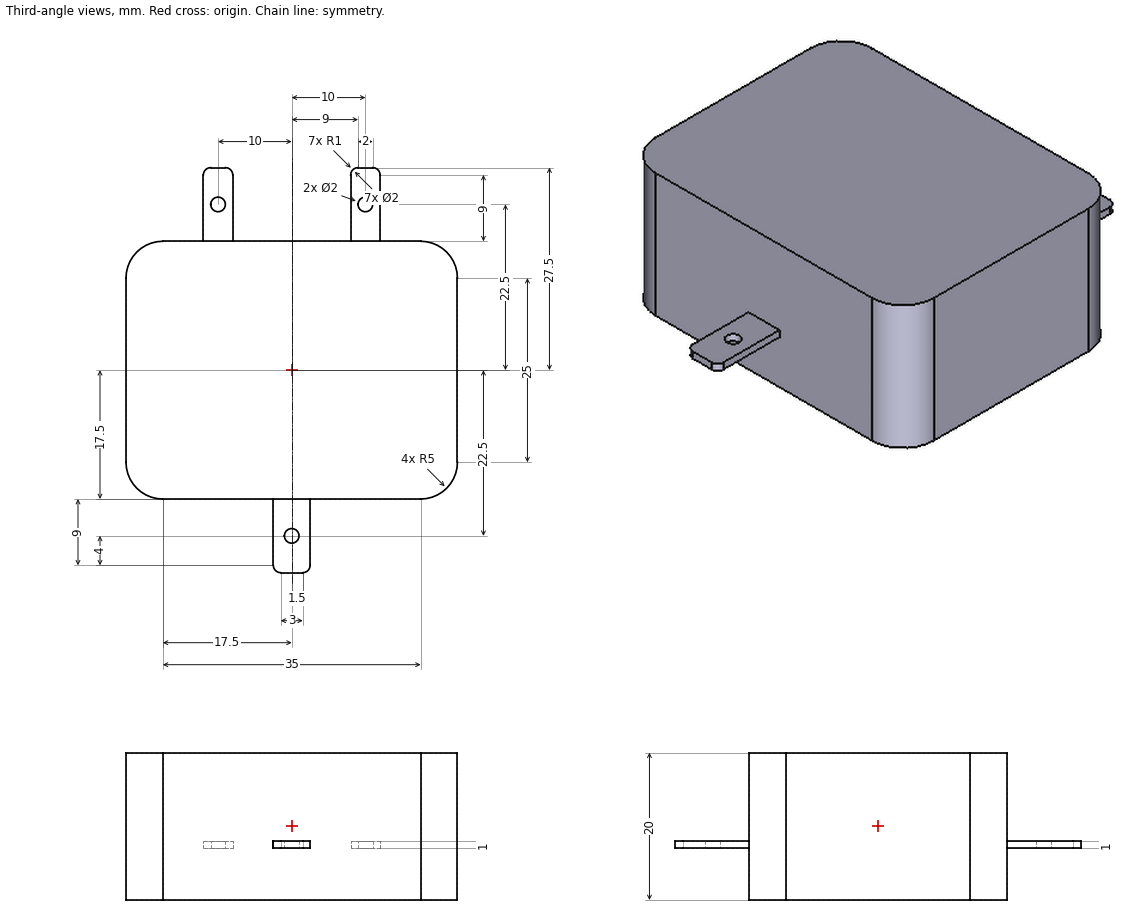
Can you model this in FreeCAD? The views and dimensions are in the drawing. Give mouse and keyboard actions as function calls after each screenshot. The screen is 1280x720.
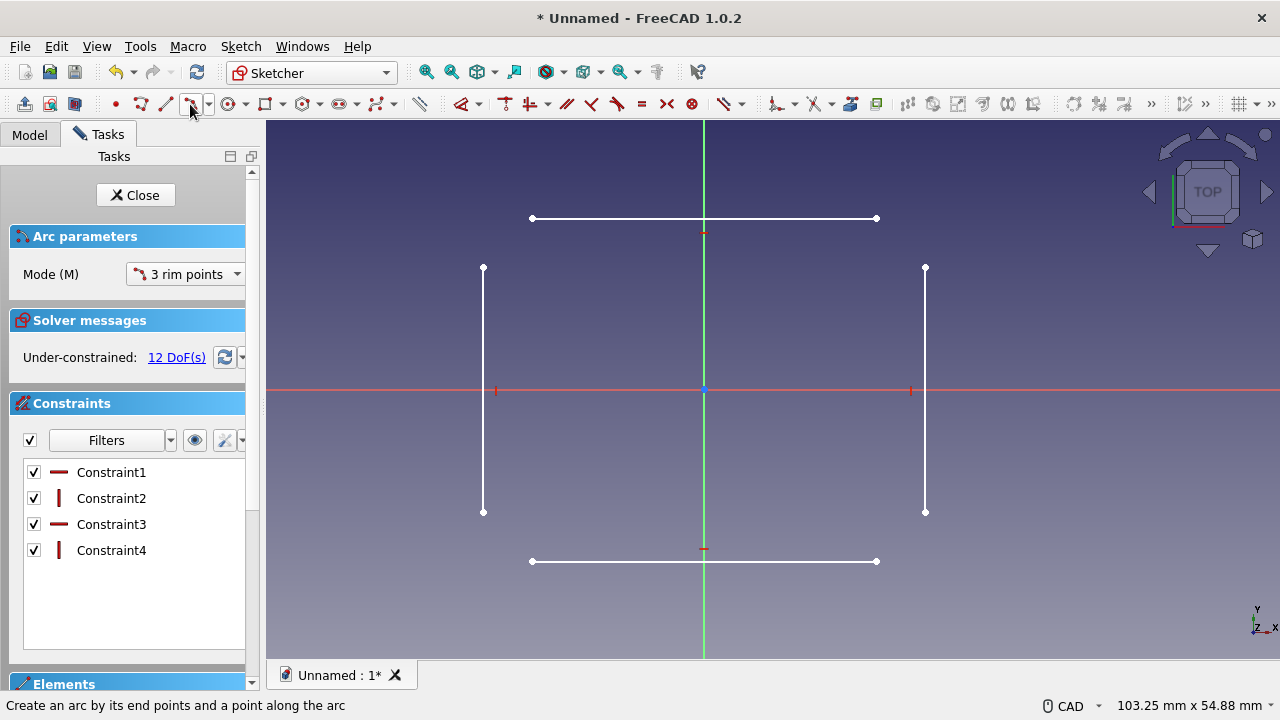
click(876, 562)
click(925, 513)
click(911, 547)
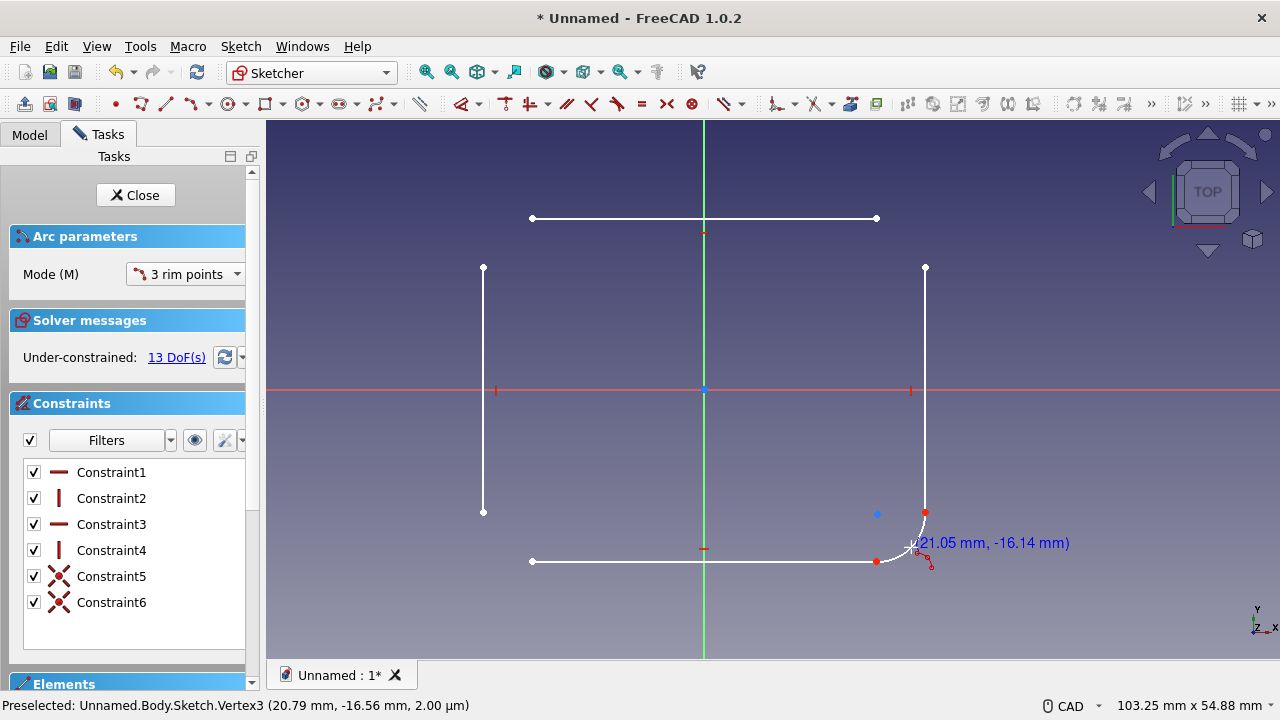
click(925, 268)
click(876, 219)
click(911, 232)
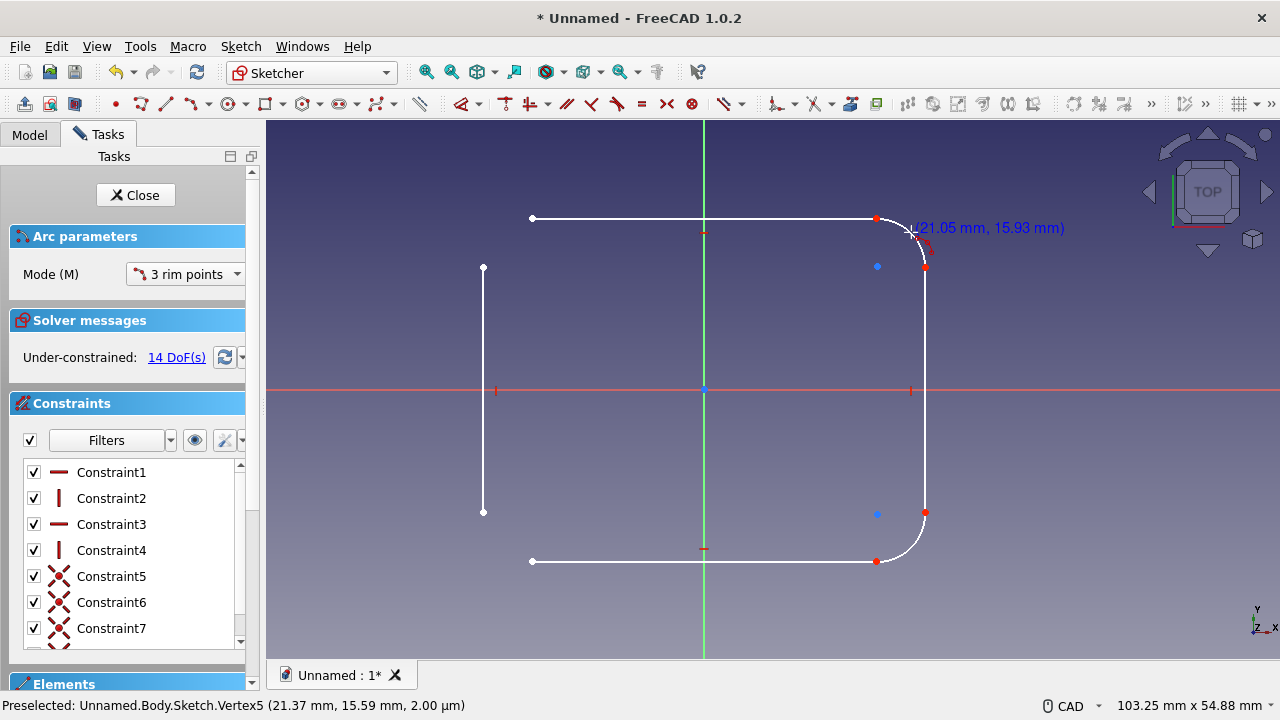
click(532, 219)
click(483, 268)
click(498, 232)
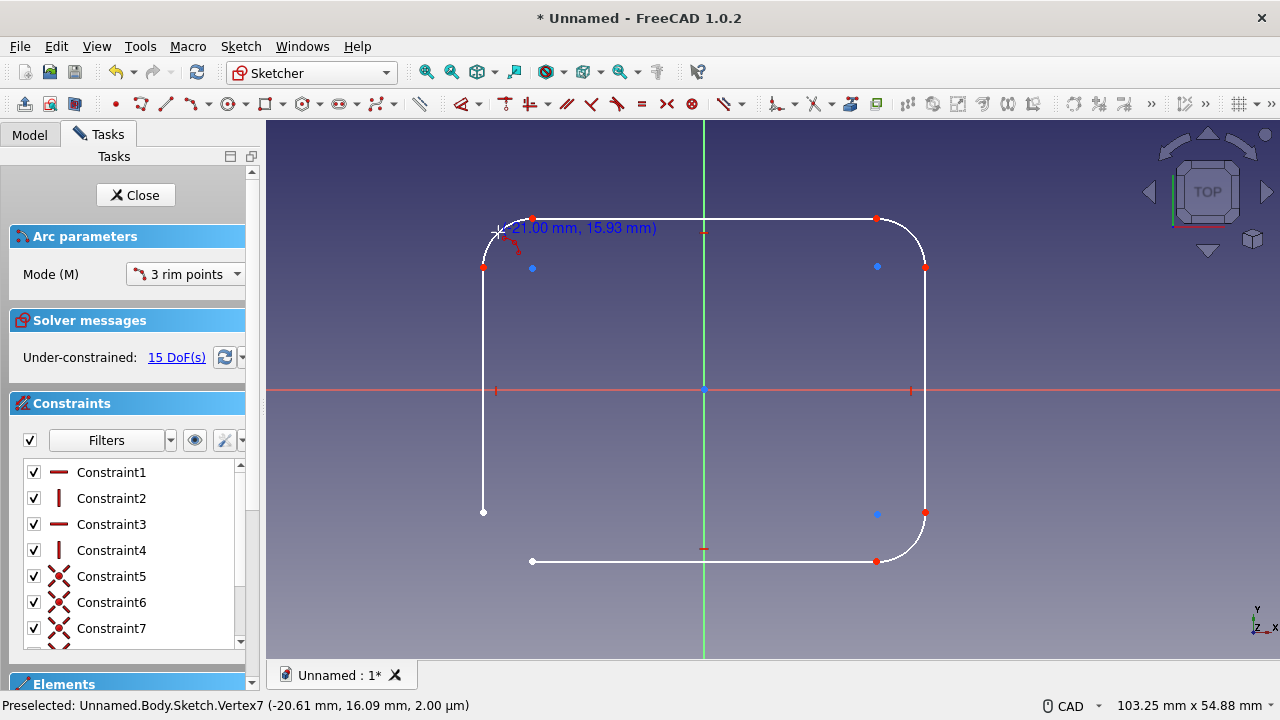
click(483, 513)
click(532, 562)
click(498, 547)
key(Escape)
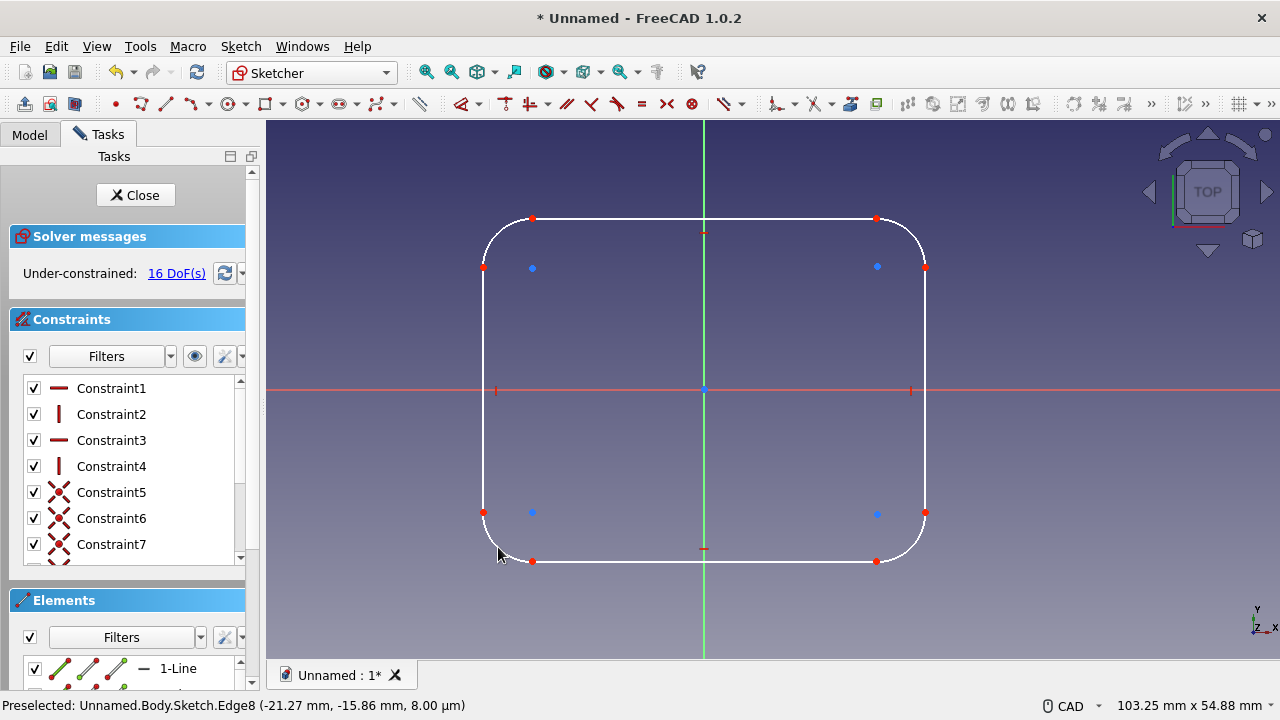
click(635, 562)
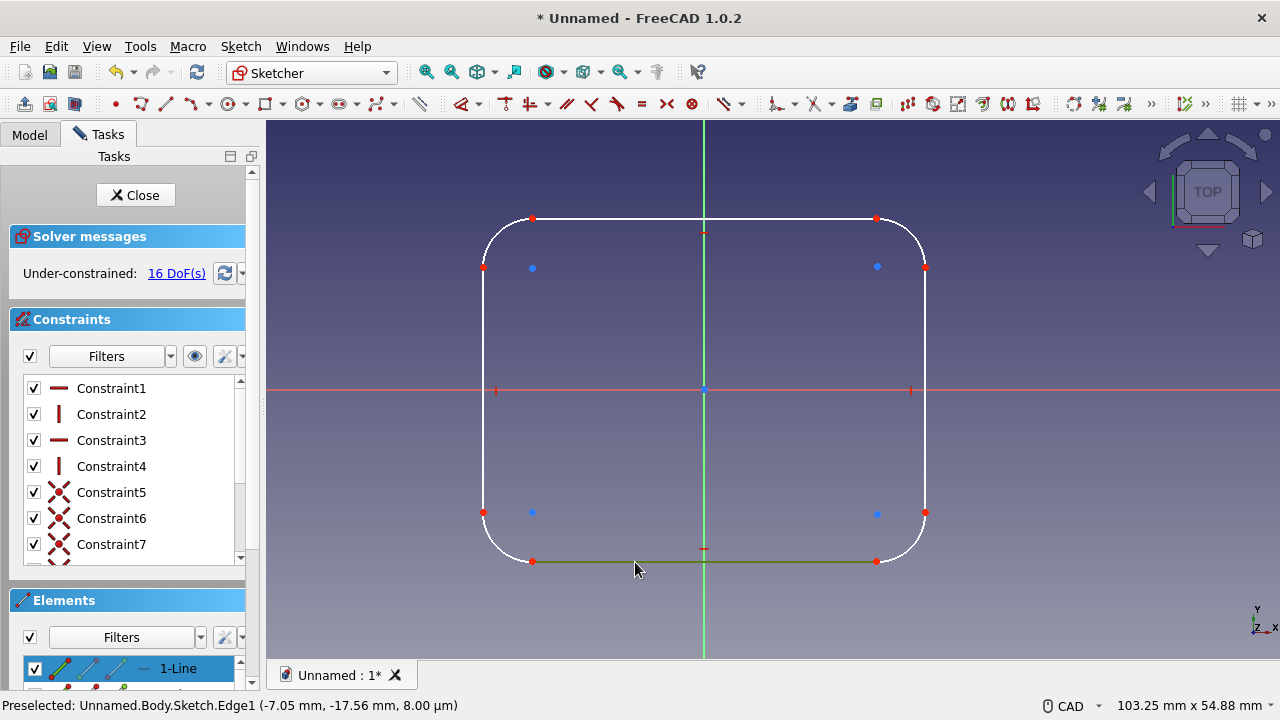
click(898, 557)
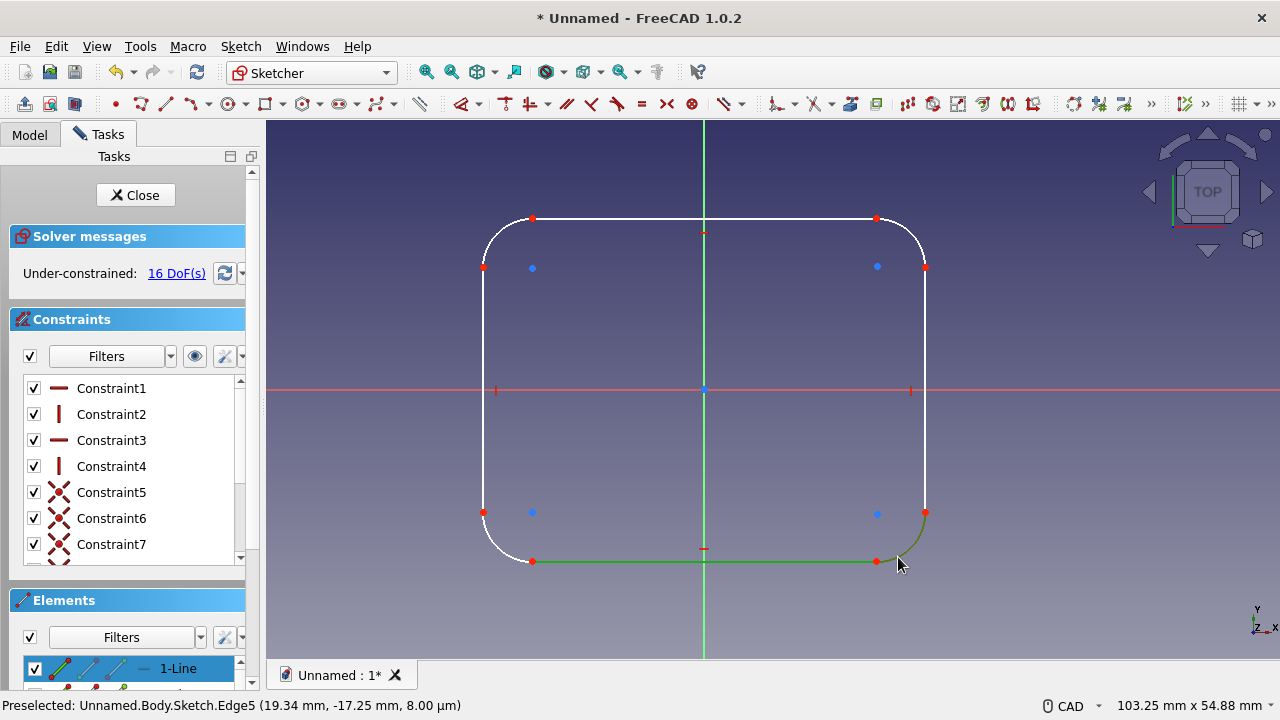
click(617, 104)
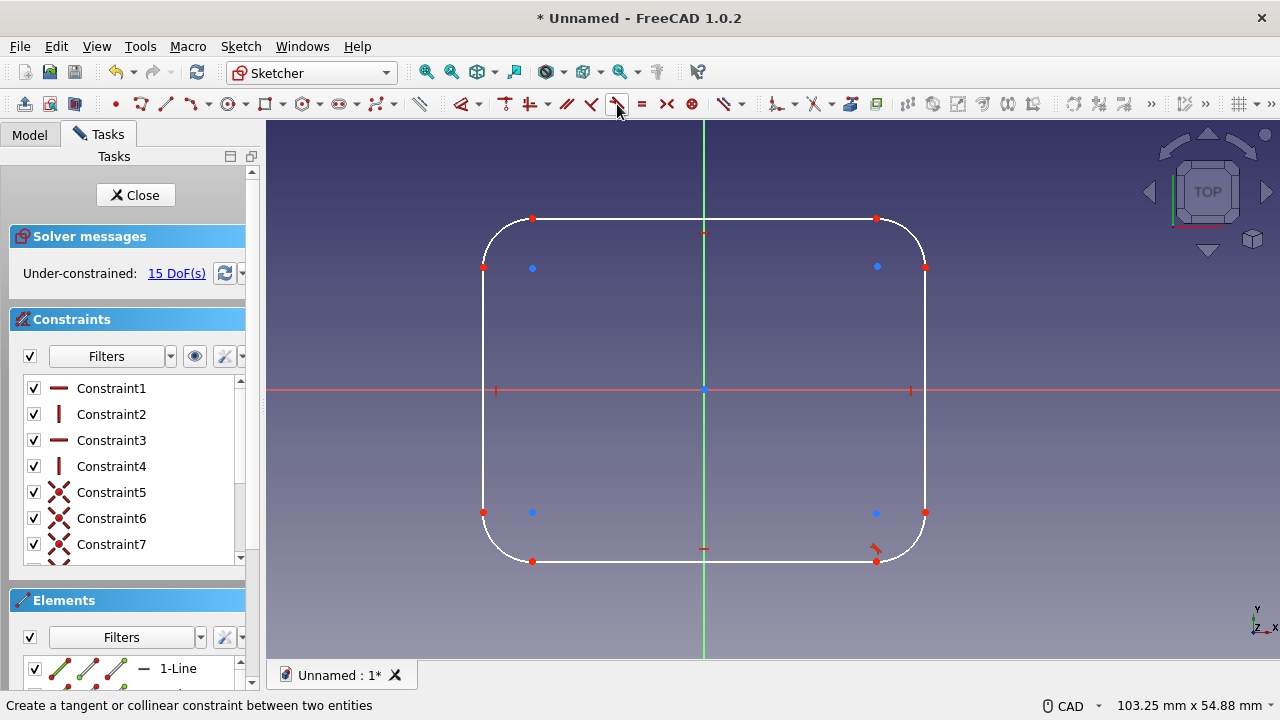
click(635, 562)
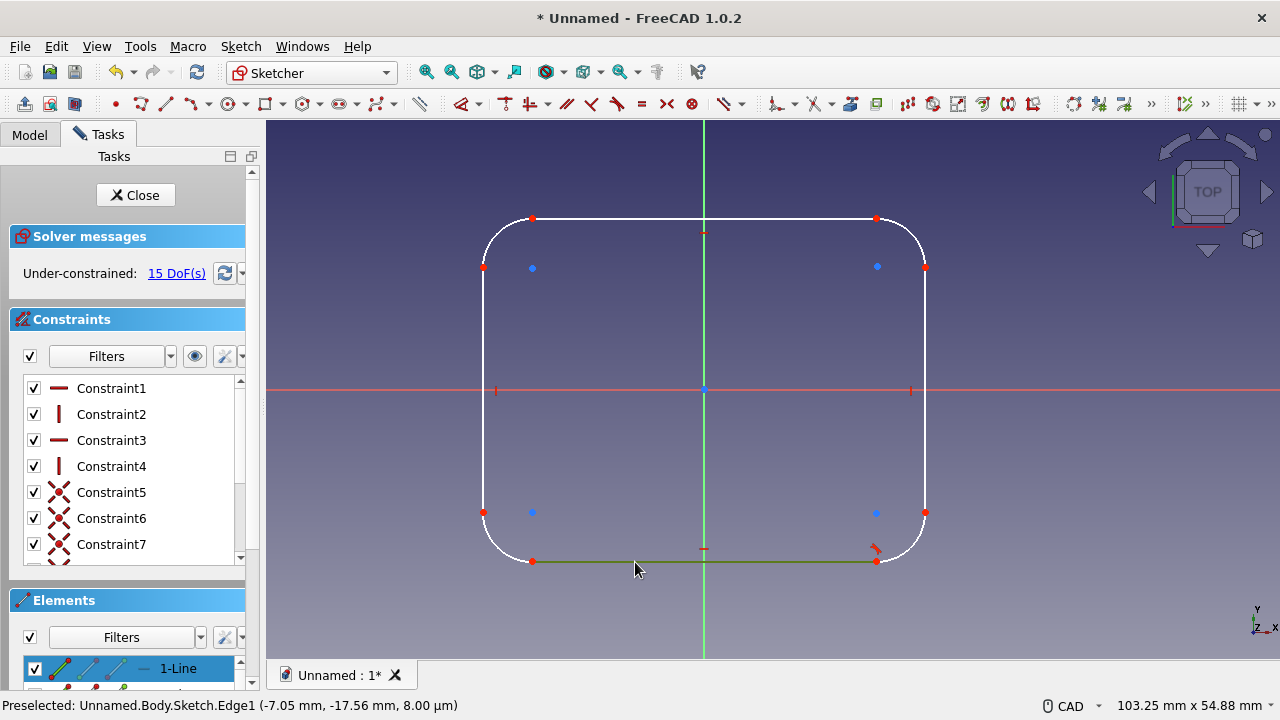
click(488, 535)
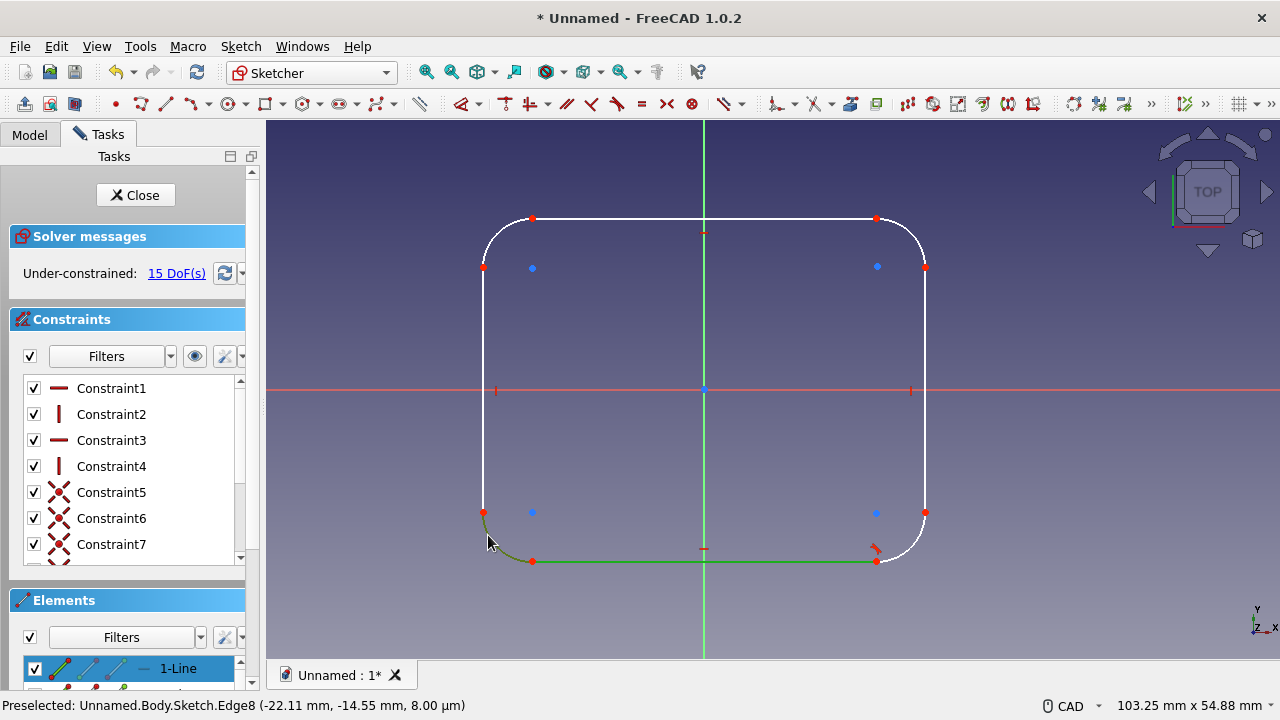
click(617, 104)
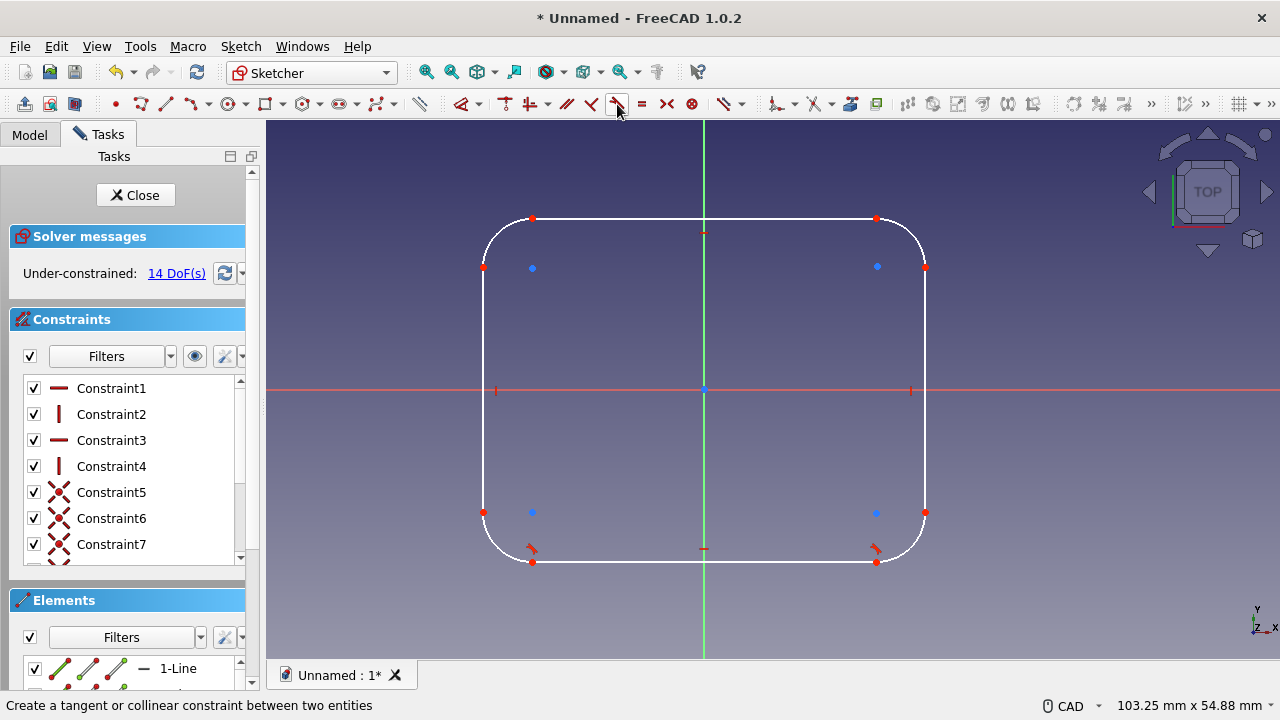
click(925, 439)